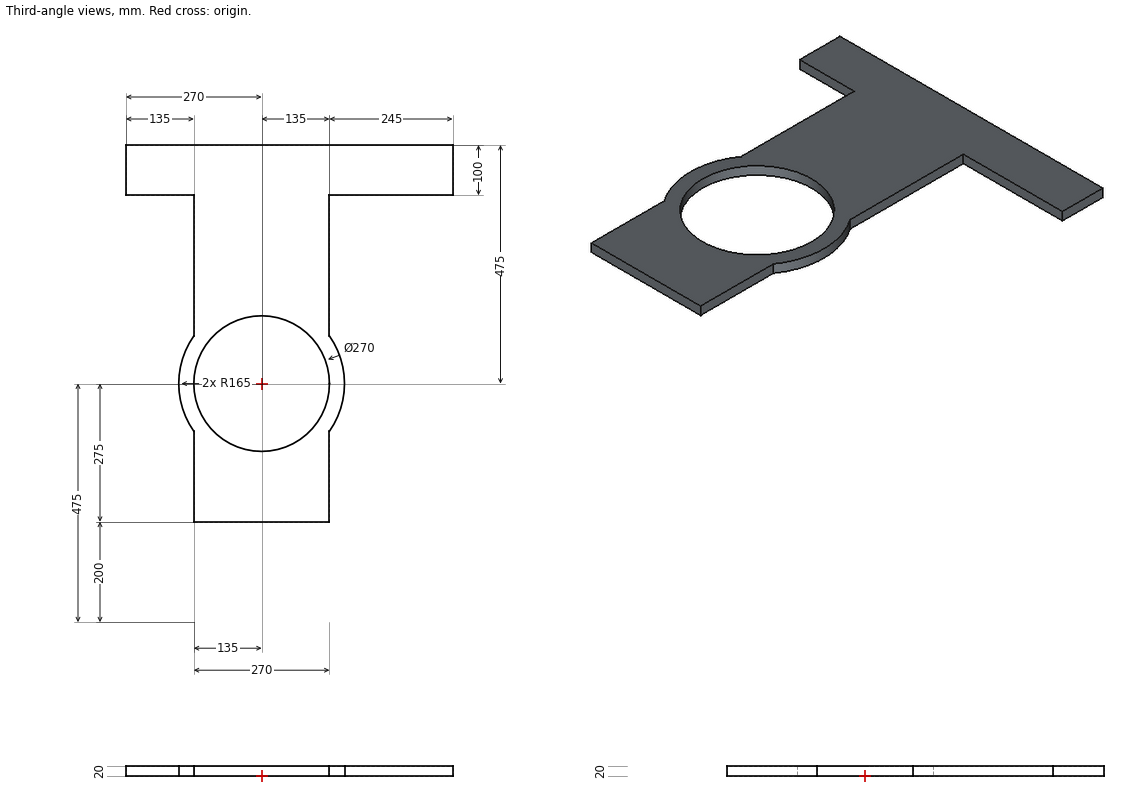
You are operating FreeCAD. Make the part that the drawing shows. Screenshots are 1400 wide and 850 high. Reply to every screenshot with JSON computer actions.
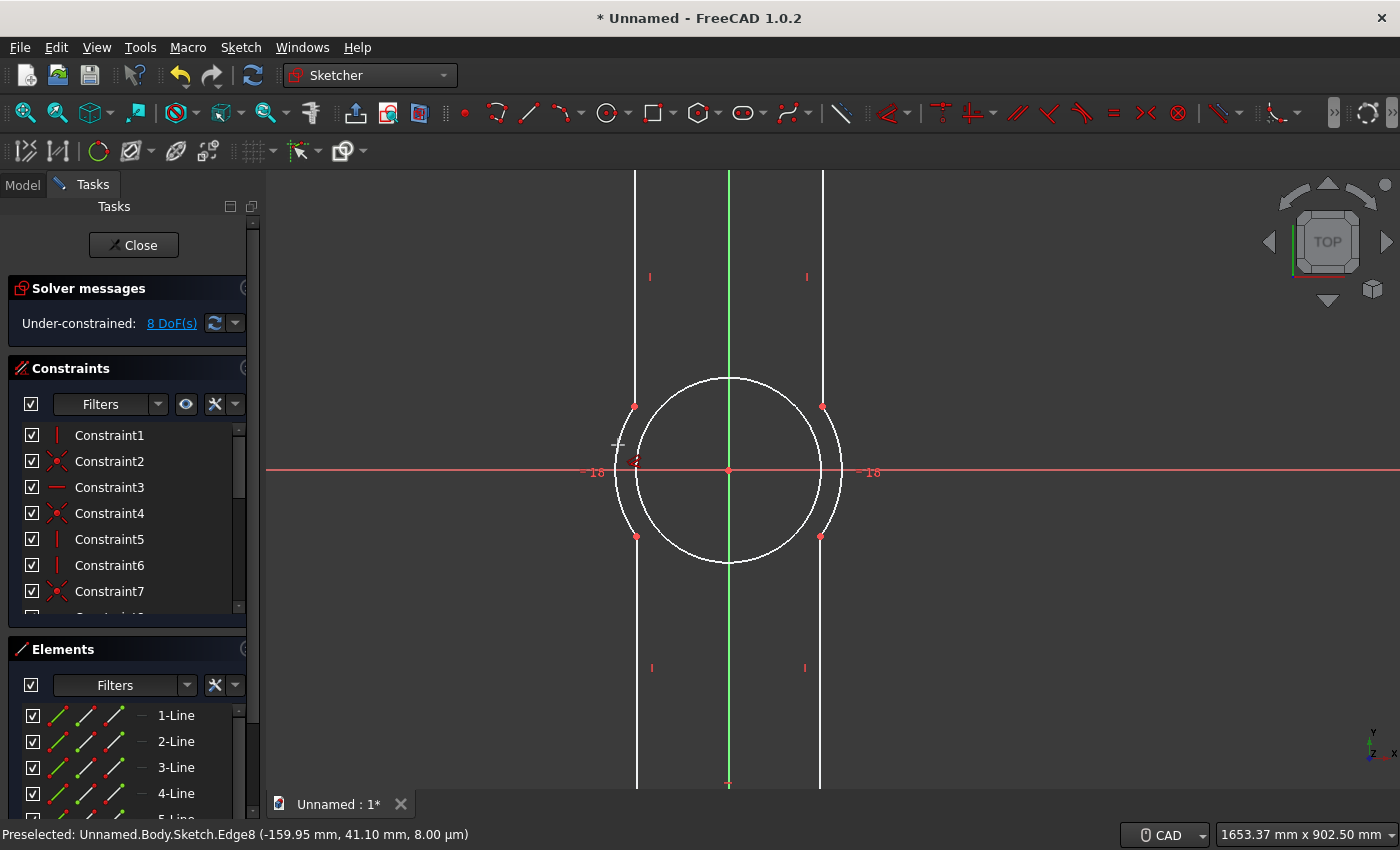
{"action": "left_click", "coordinate": [838, 499]}
{"action": "left_click", "coordinate": [869, 507]}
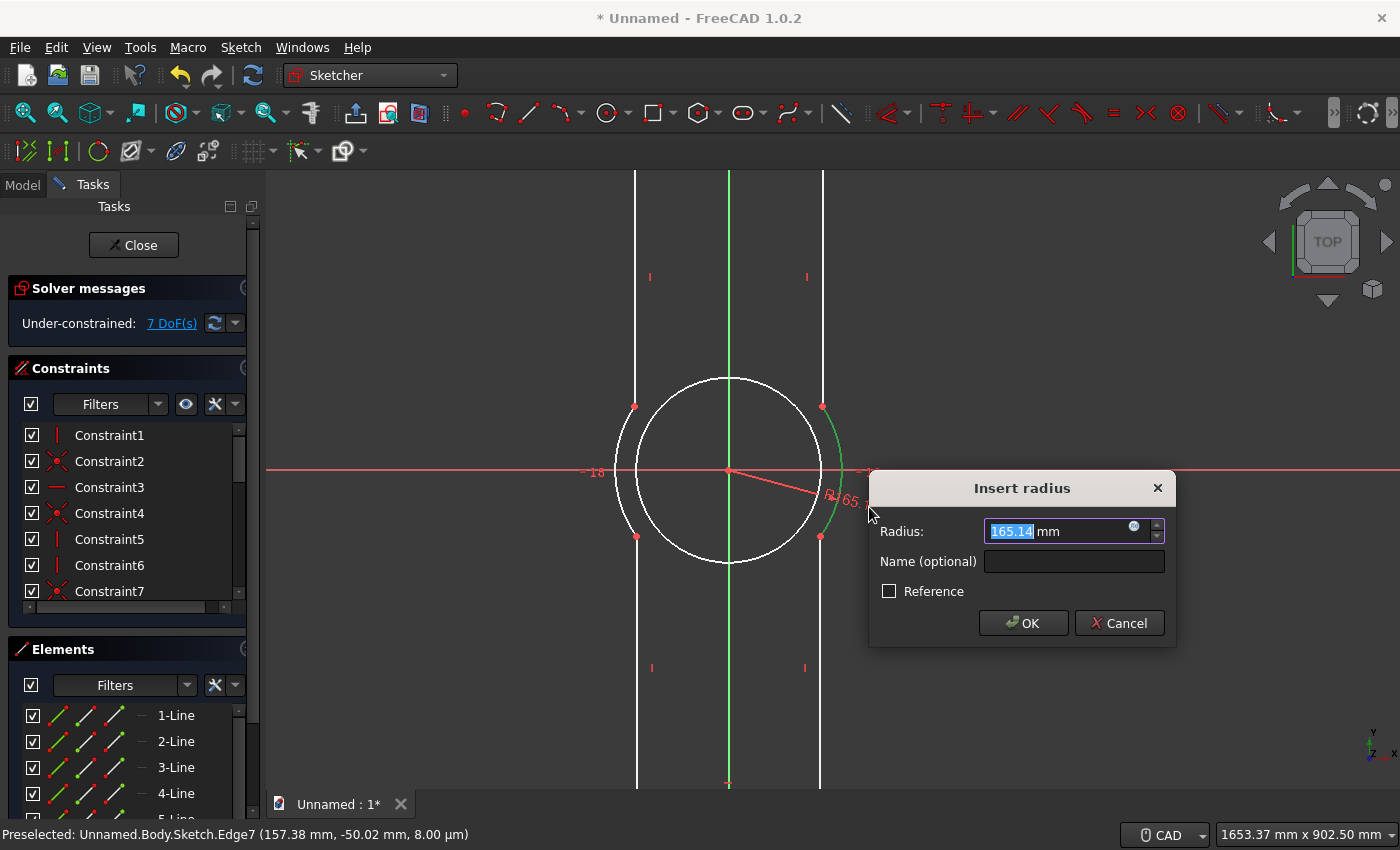
{"action": "type", "text": "165"}
{"action": "key", "text": "Return"}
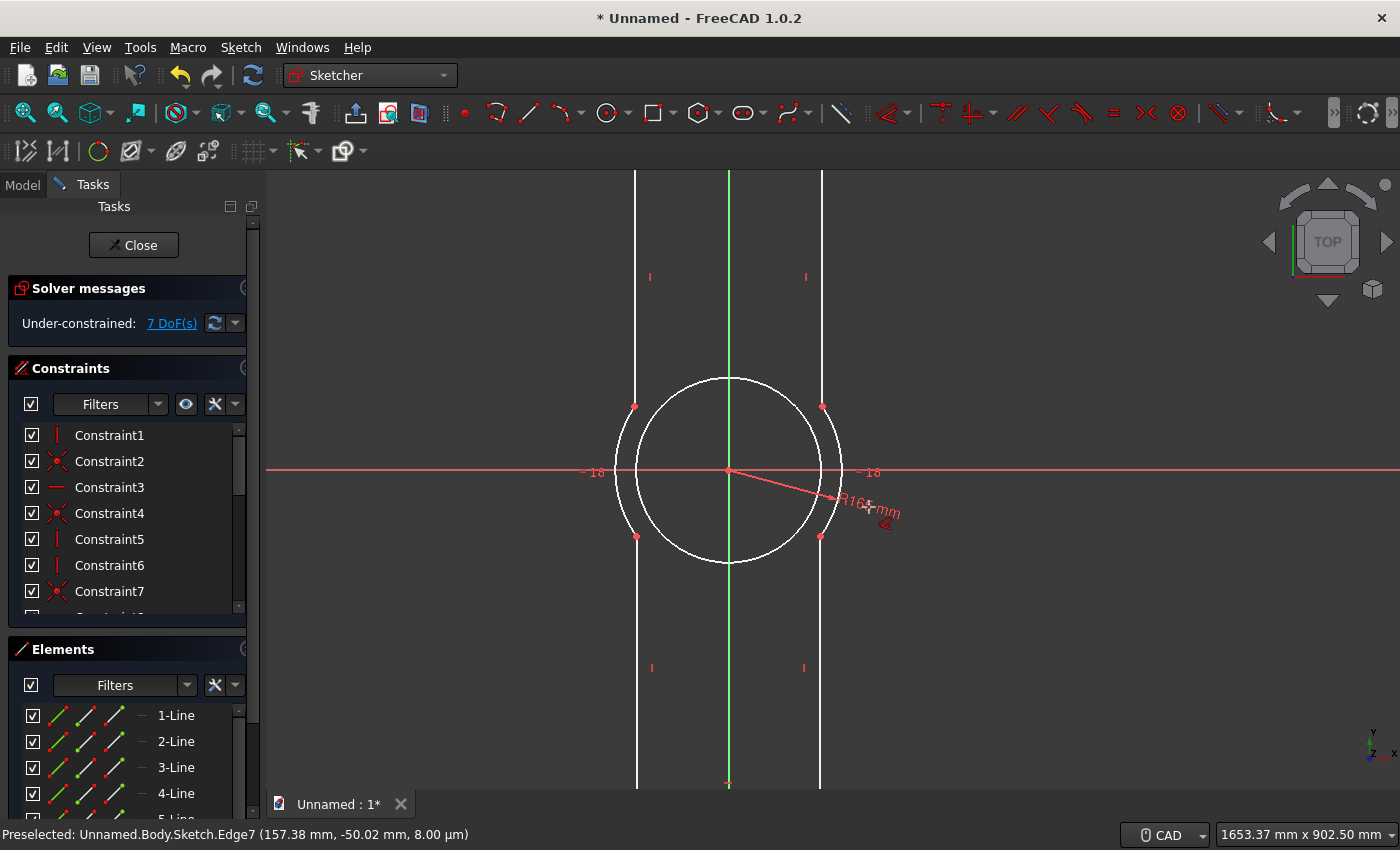
{"action": "left_click", "coordinate": [794, 405]}
{"action": "left_click", "coordinate": [764, 351]}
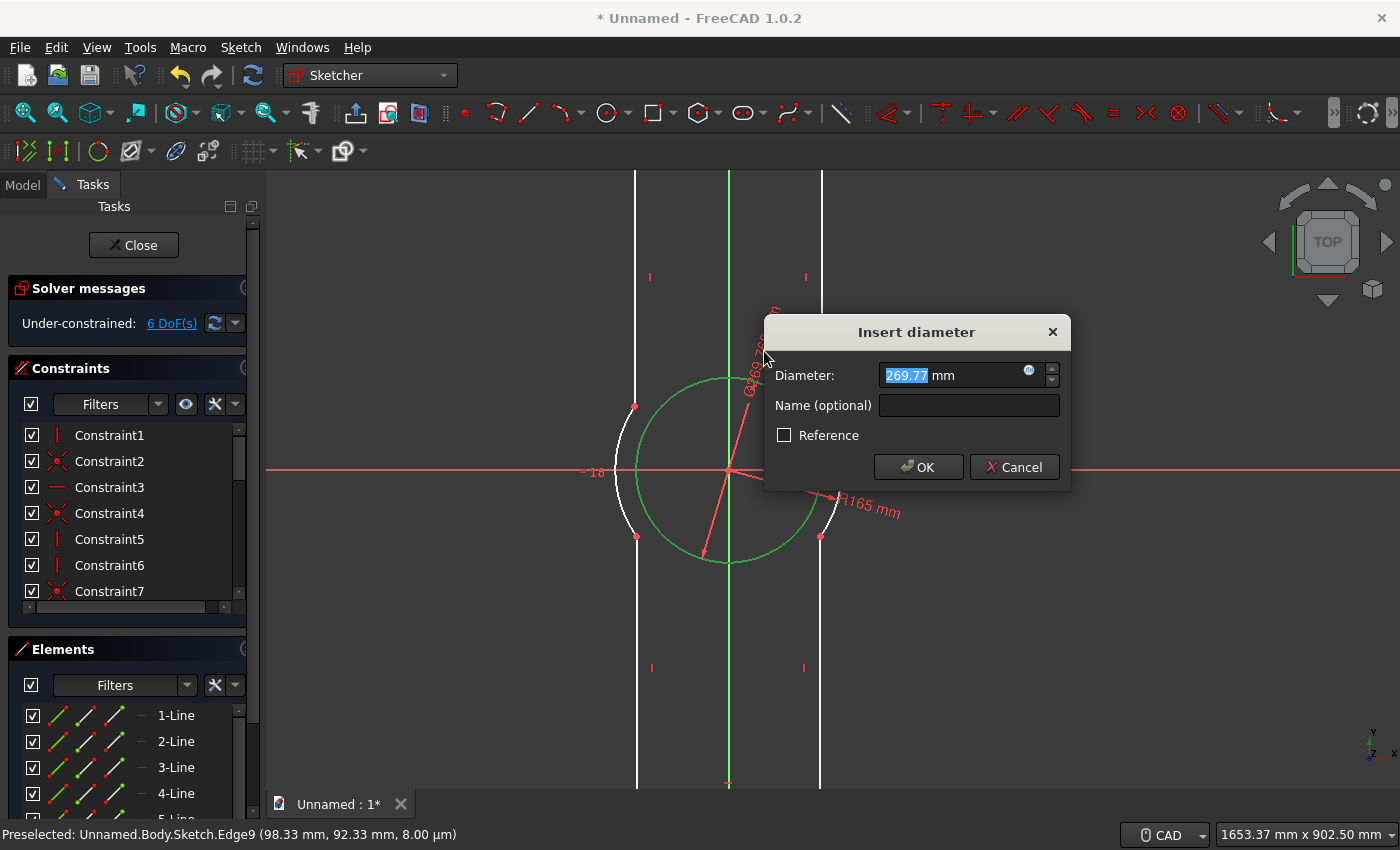
{"action": "type", "text": "270"}
{"action": "key", "text": "Return"}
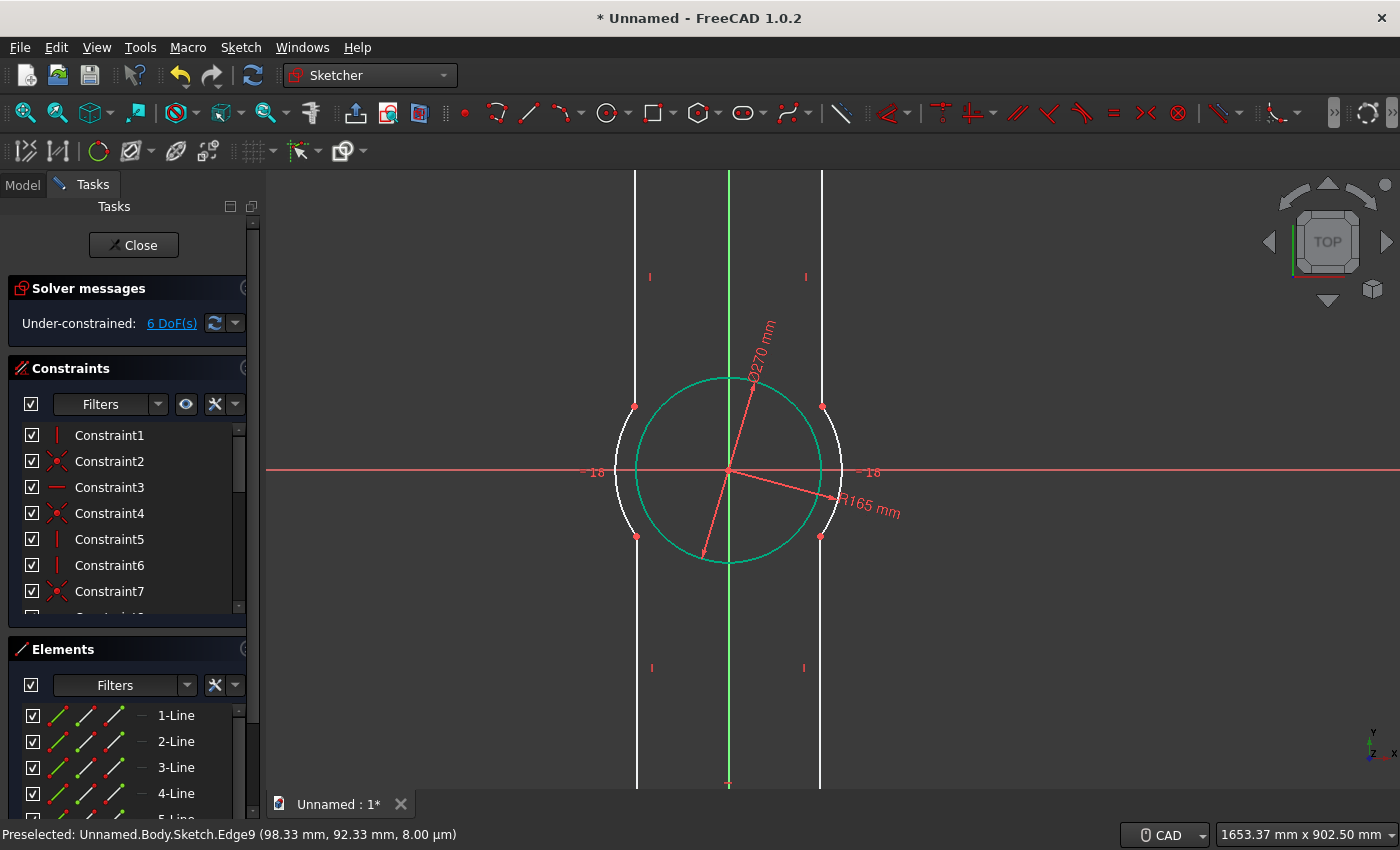
{"action": "scroll", "coordinate": [838, 498], "scroll_direction": "down", "scroll_amount": 2}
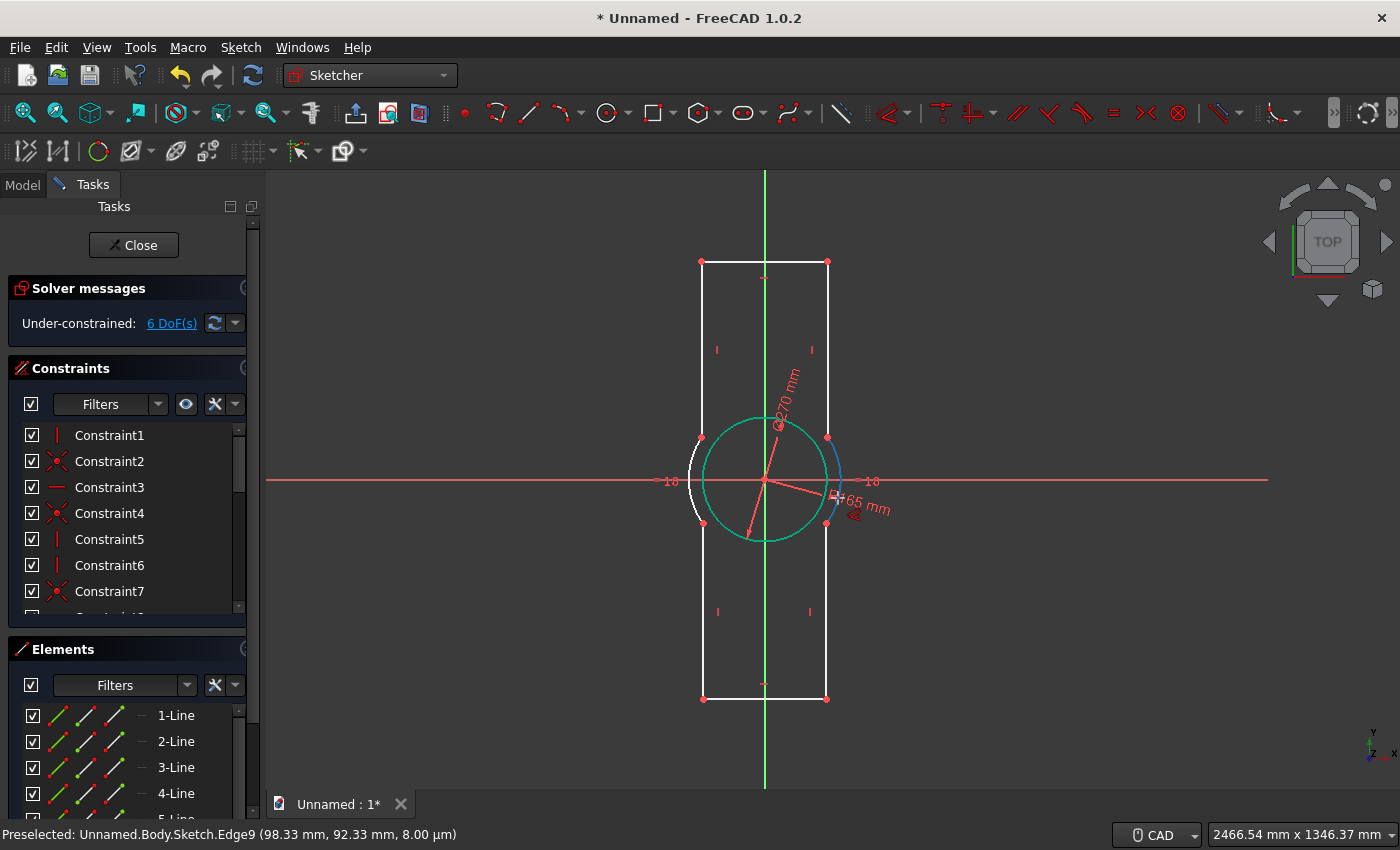
{"action": "left_click", "coordinate": [740, 699]}
{"action": "left_click", "coordinate": [736, 733]}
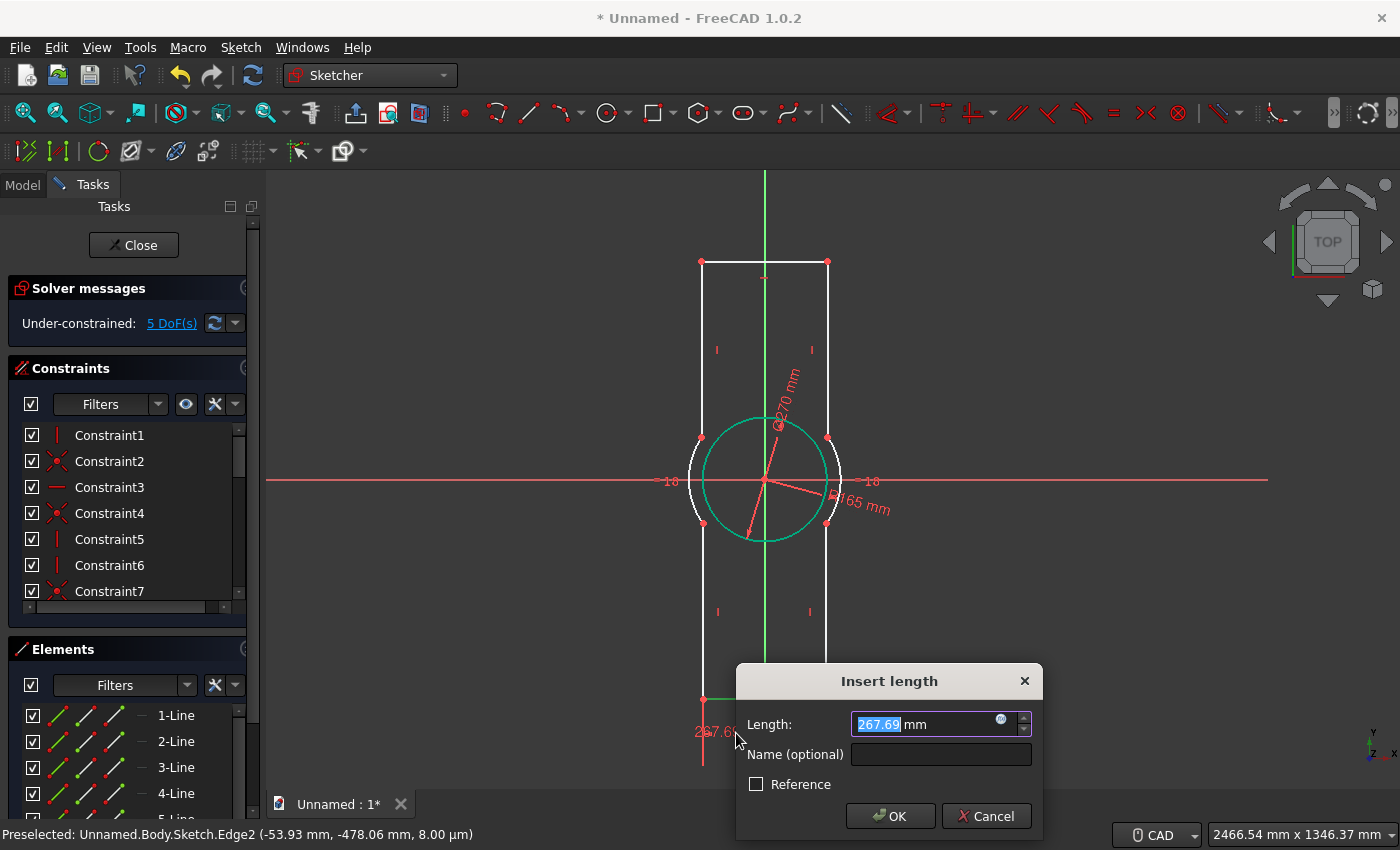
{"action": "type", "text": "270"}
{"action": "key", "text": "Return"}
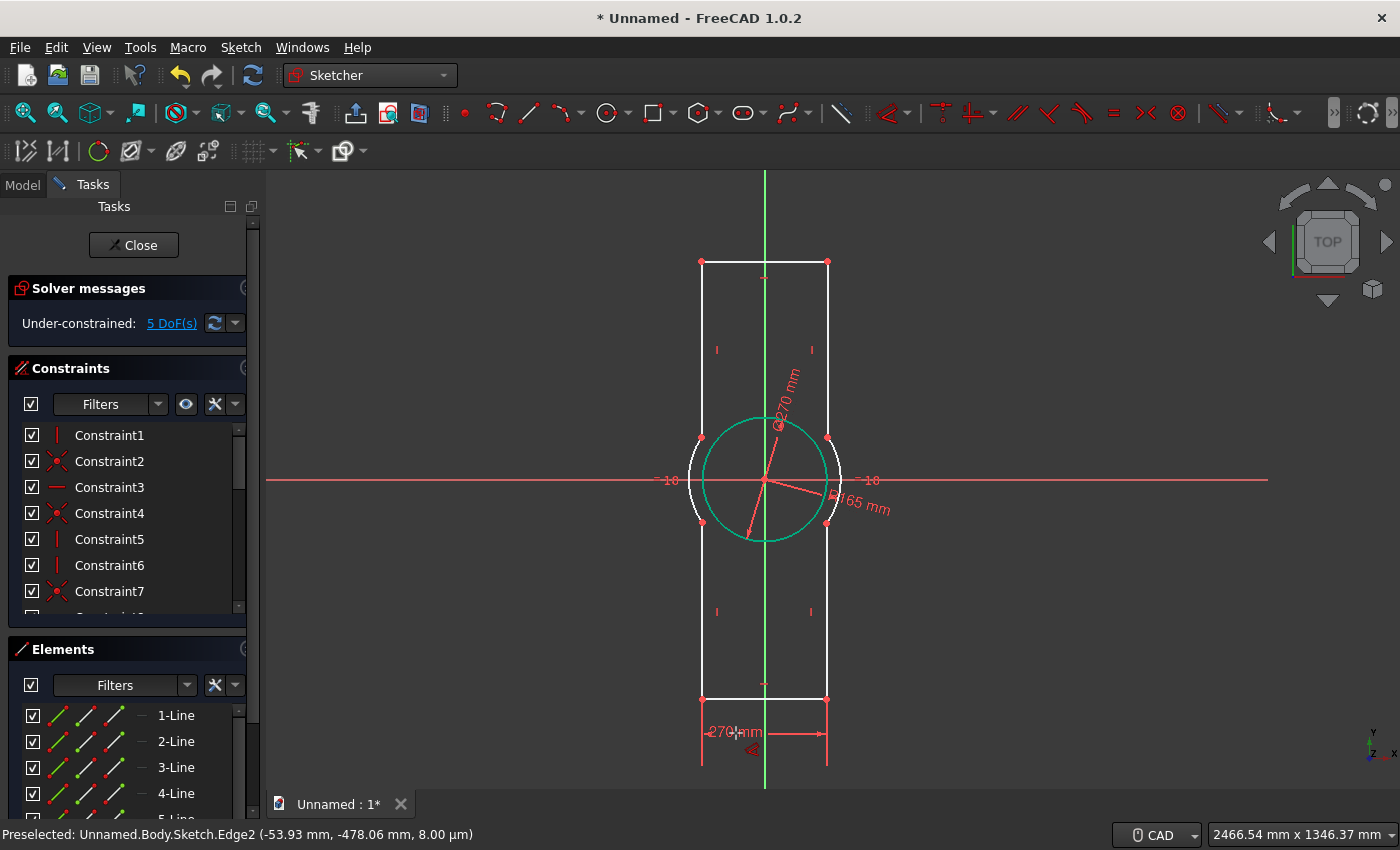
{"action": "left_click", "coordinate": [790, 262]}
{"action": "left_click", "coordinate": [736, 228]}